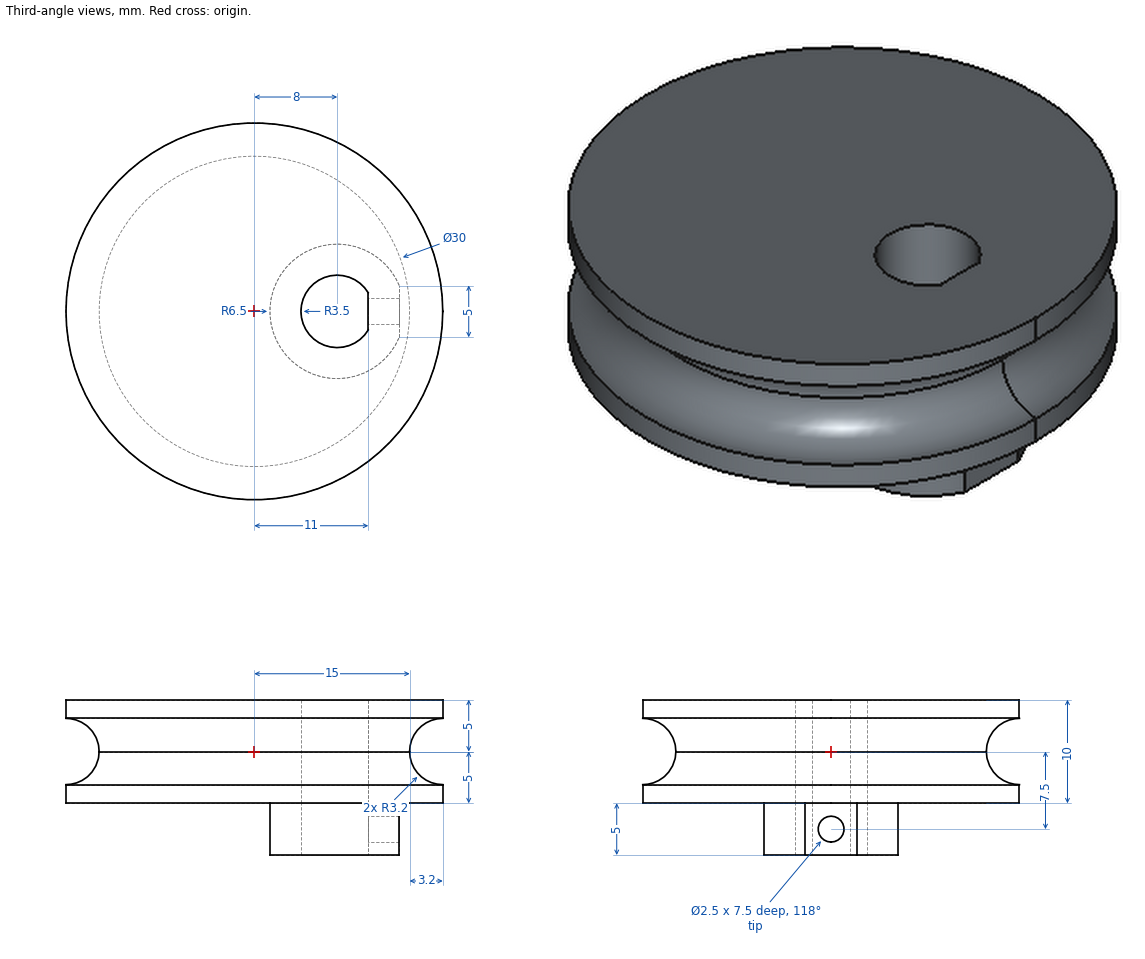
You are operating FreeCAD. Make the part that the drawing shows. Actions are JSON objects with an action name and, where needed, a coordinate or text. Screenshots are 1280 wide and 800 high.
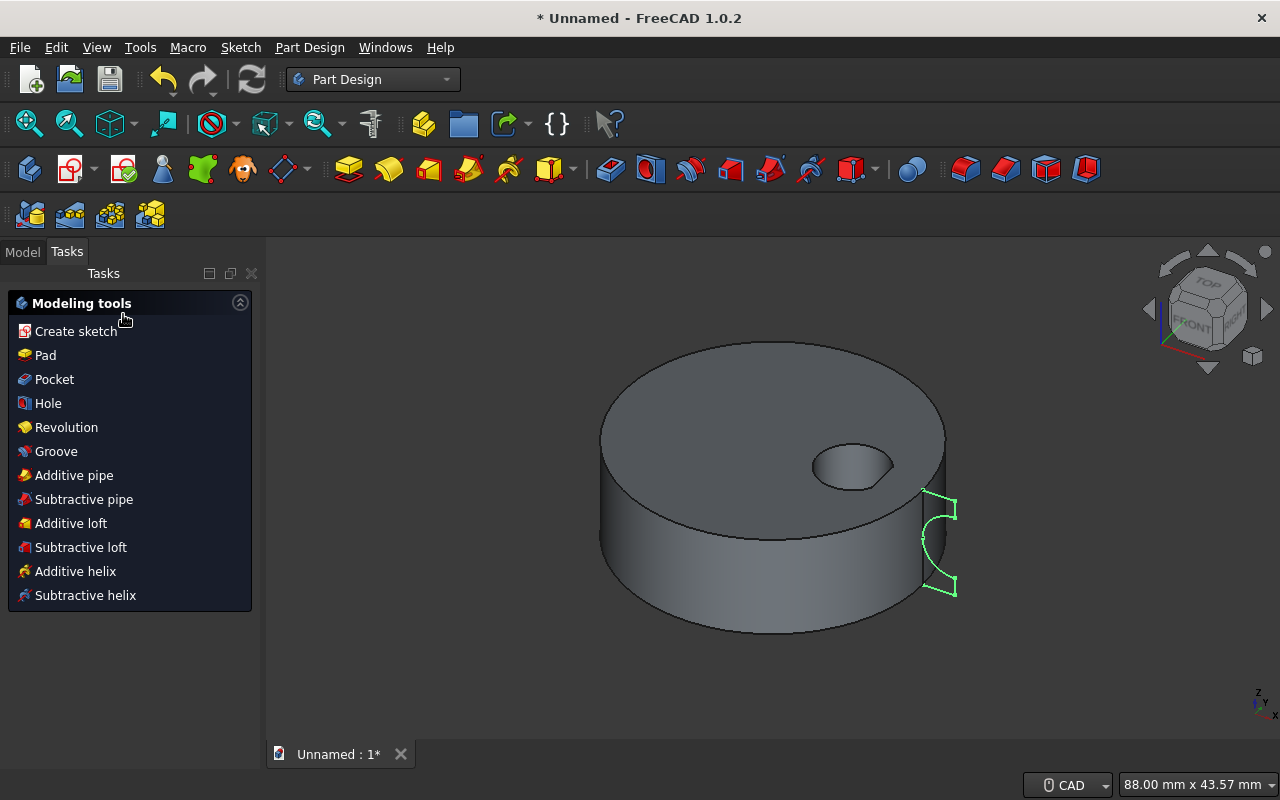
{"action": "left_click", "coordinate": [390, 170]}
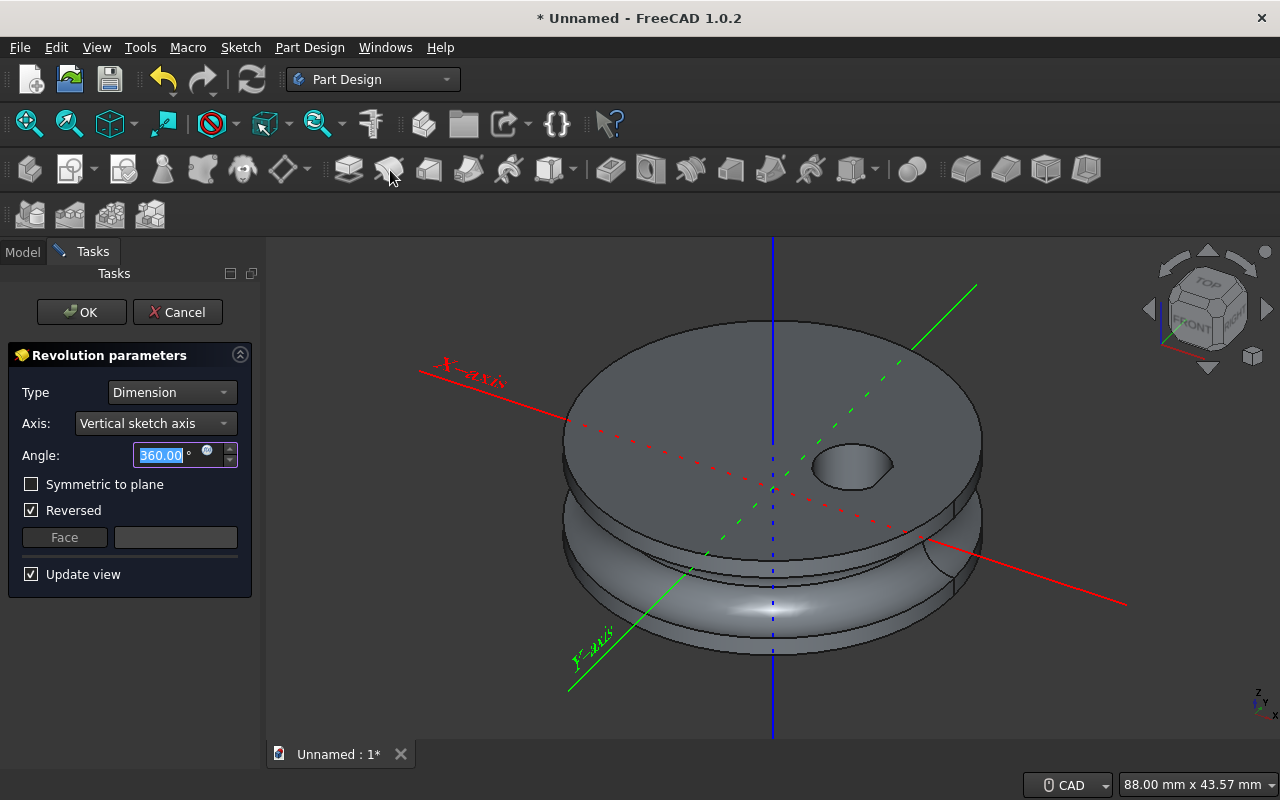
{"action": "left_click", "coordinate": [82, 312]}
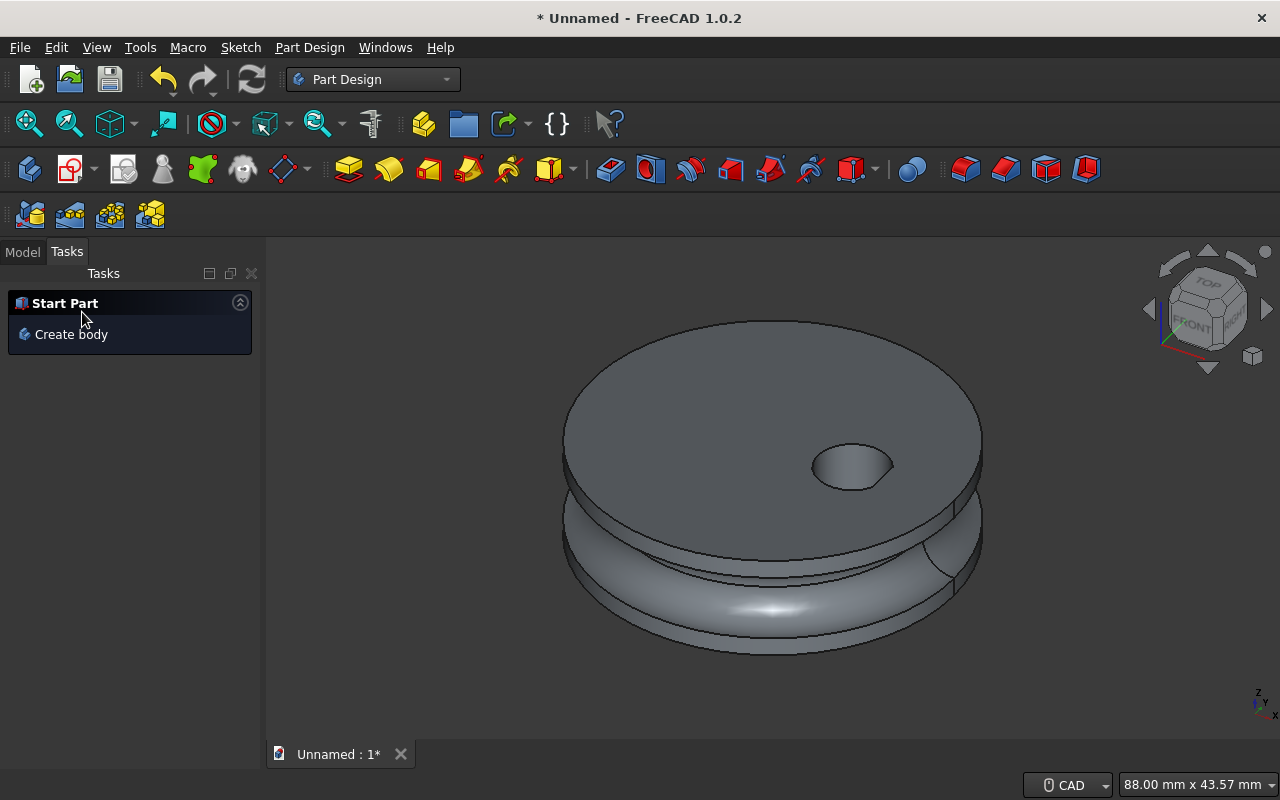
{"action": "key", "text": "5"}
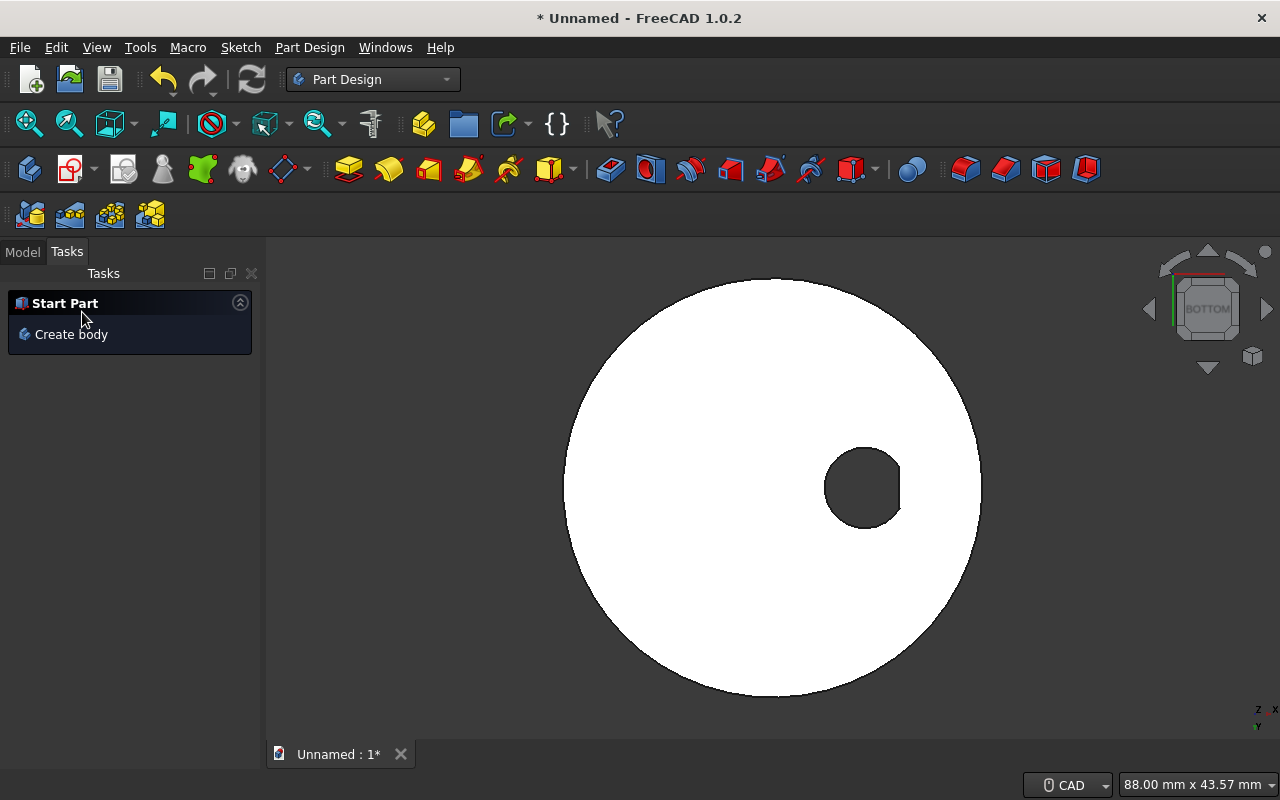
{"action": "left_click", "coordinate": [713, 547]}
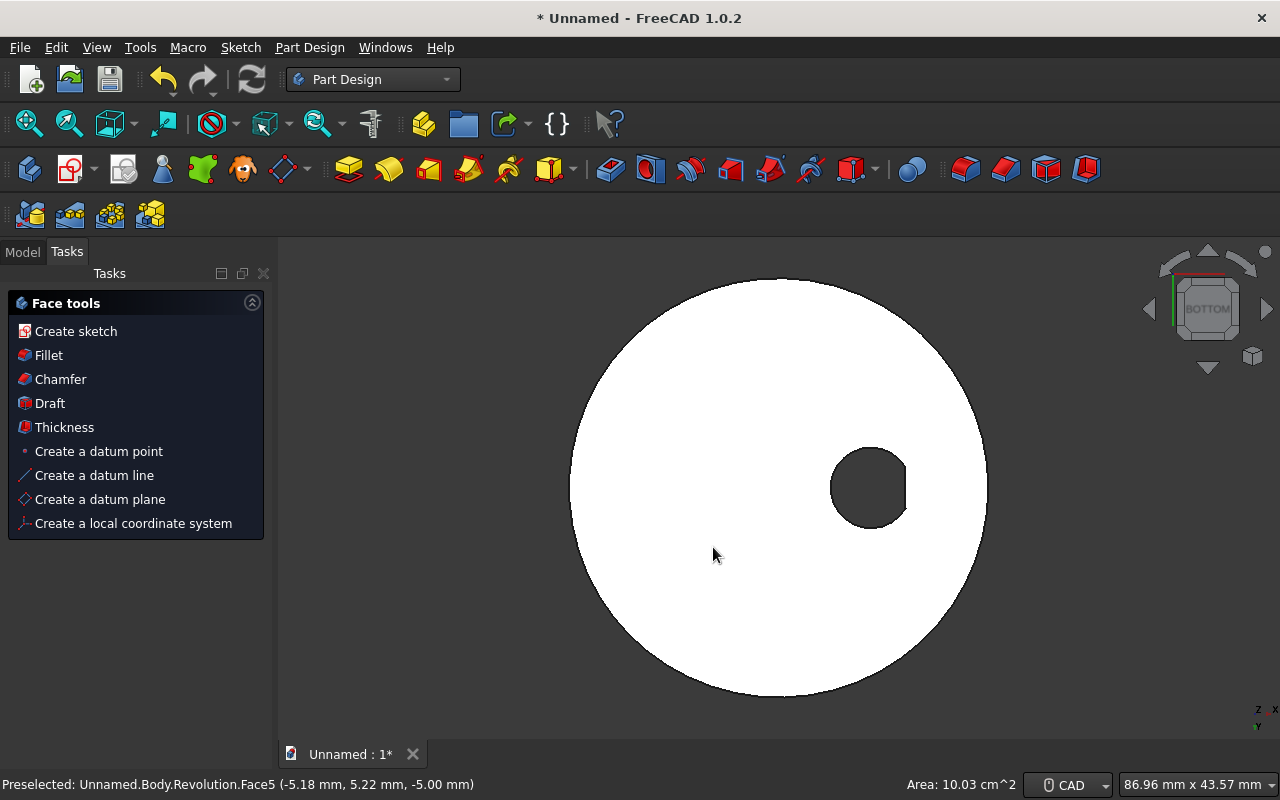
{"action": "left_click", "coordinate": [70, 170]}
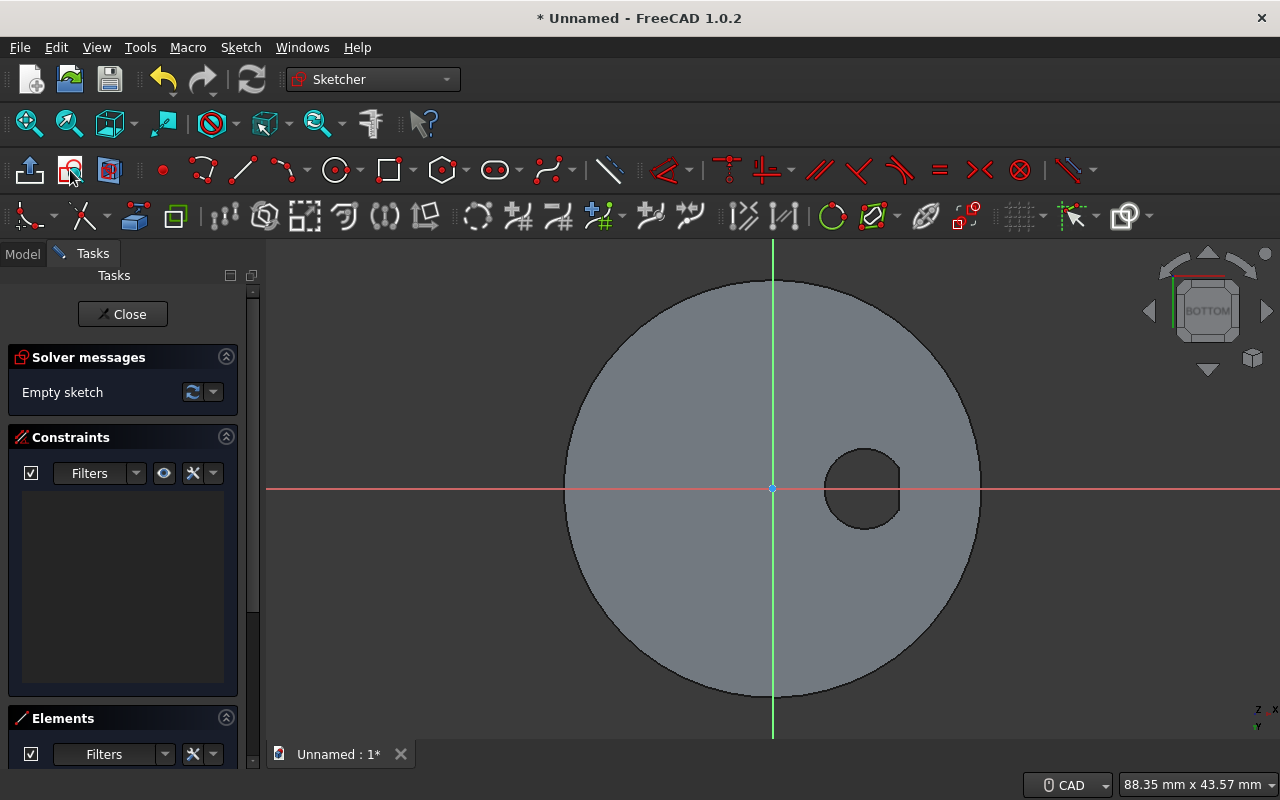
{"action": "scroll", "coordinate": [917, 489], "scroll_direction": "up", "scroll_amount": 6}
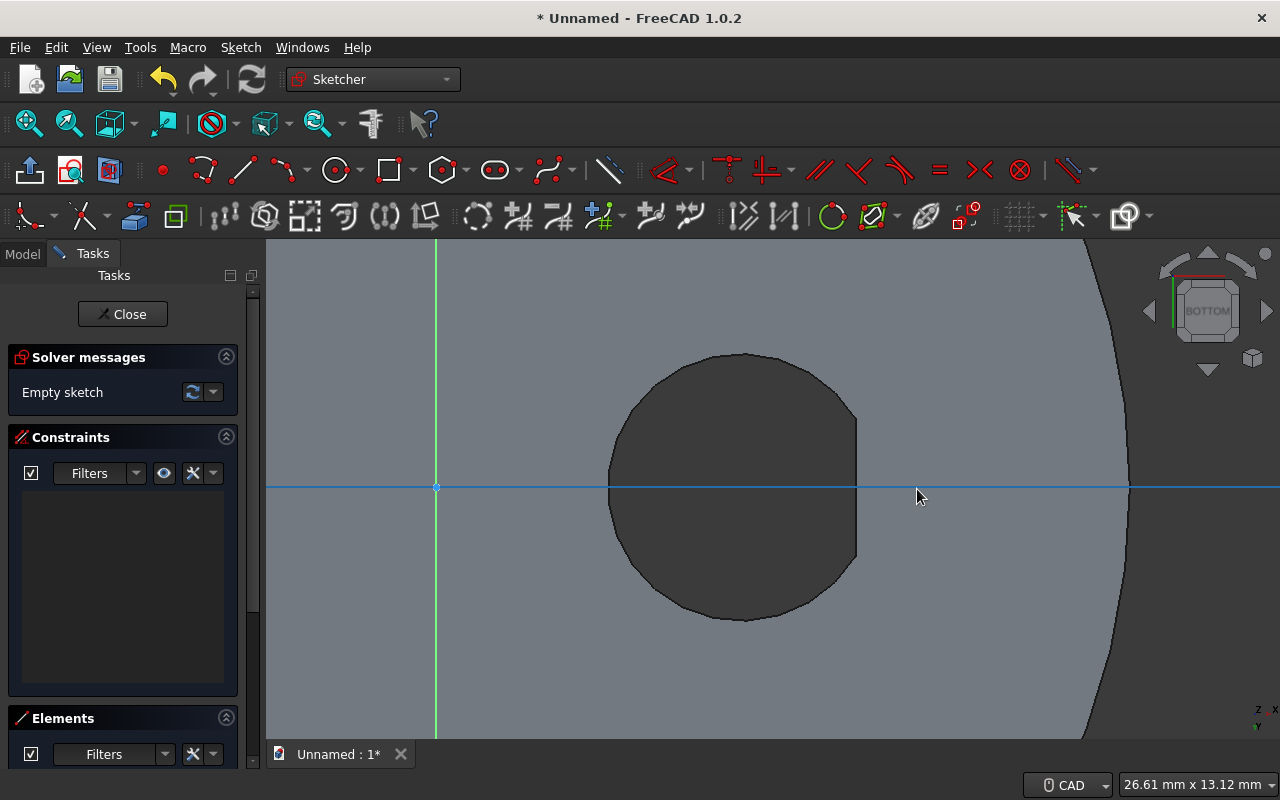
{"action": "left_click", "coordinate": [244, 170]}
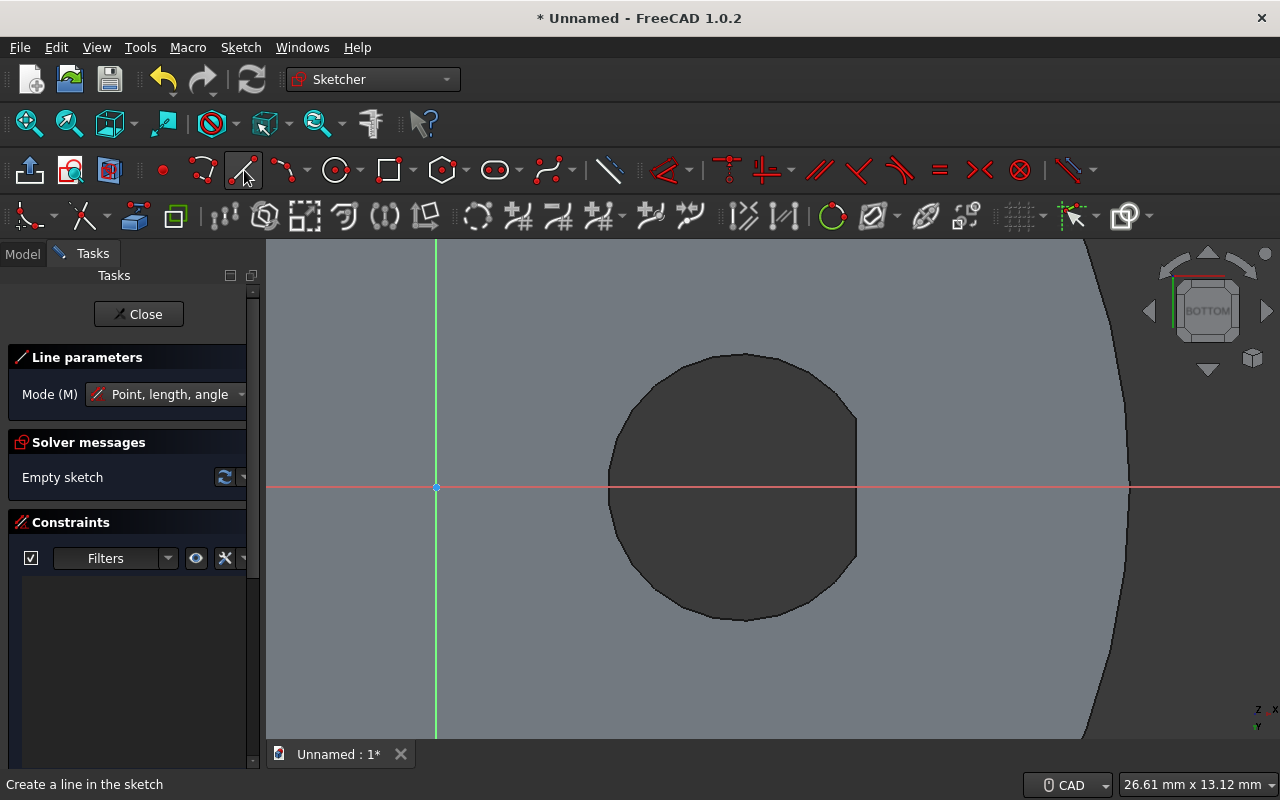
{"action": "left_click", "coordinate": [970, 392]}
{"action": "left_click", "coordinate": [970, 583]}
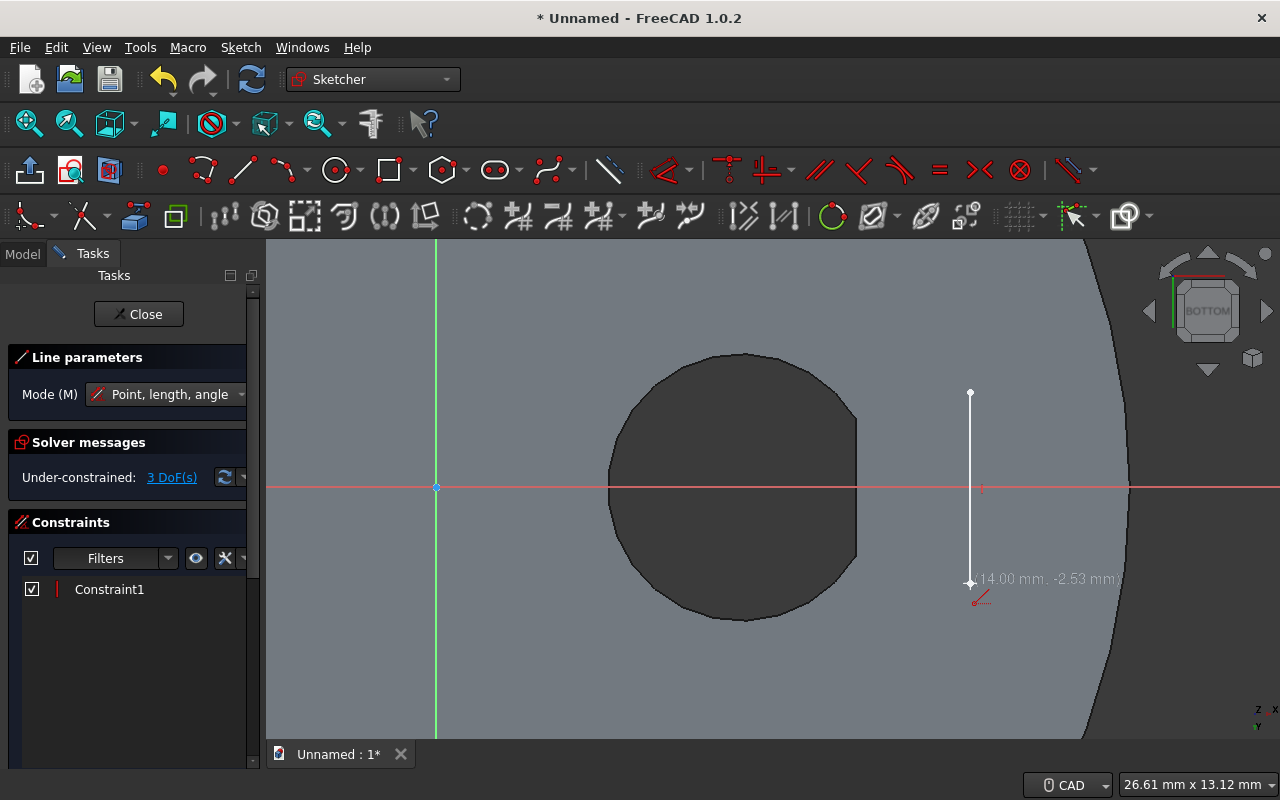
{"action": "left_click", "coordinate": [284, 170]}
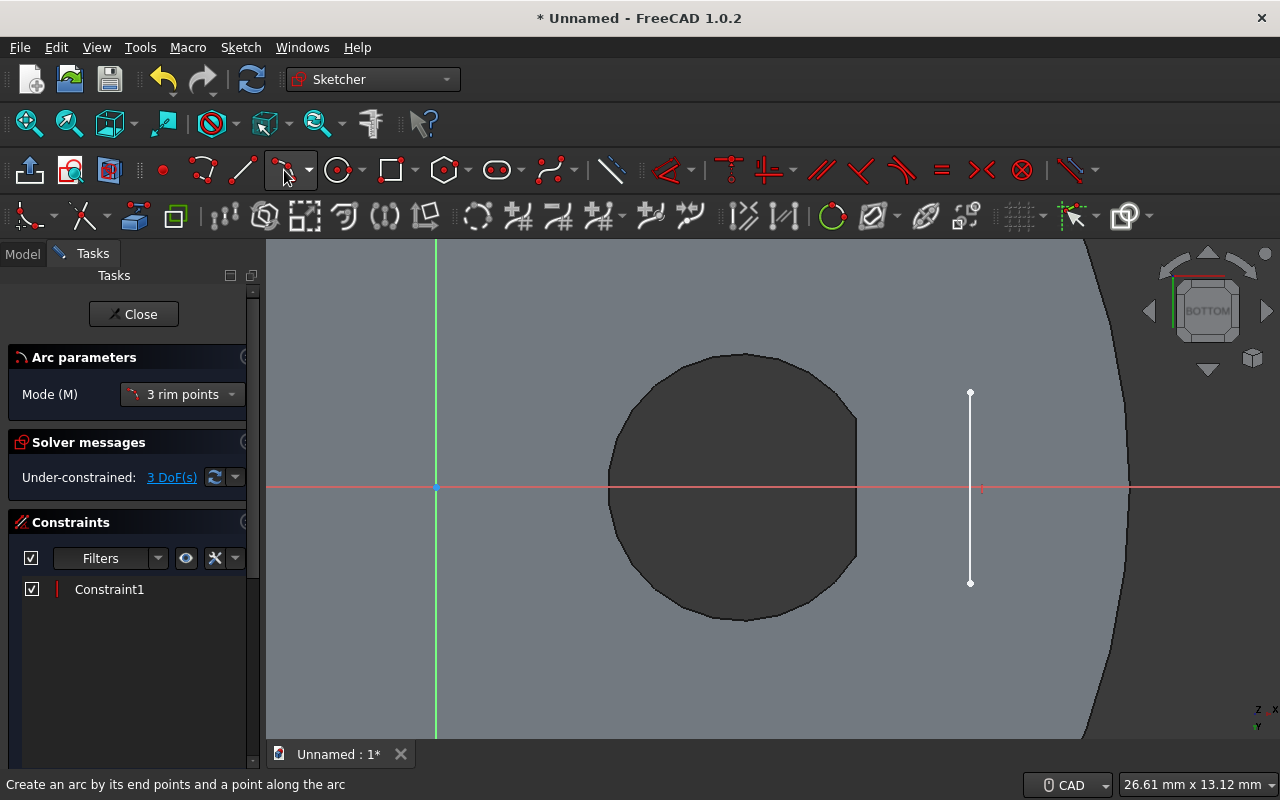
{"action": "left_click", "coordinate": [970, 584]}
{"action": "left_click", "coordinate": [970, 393]}
{"action": "left_click", "coordinate": [530, 358]}